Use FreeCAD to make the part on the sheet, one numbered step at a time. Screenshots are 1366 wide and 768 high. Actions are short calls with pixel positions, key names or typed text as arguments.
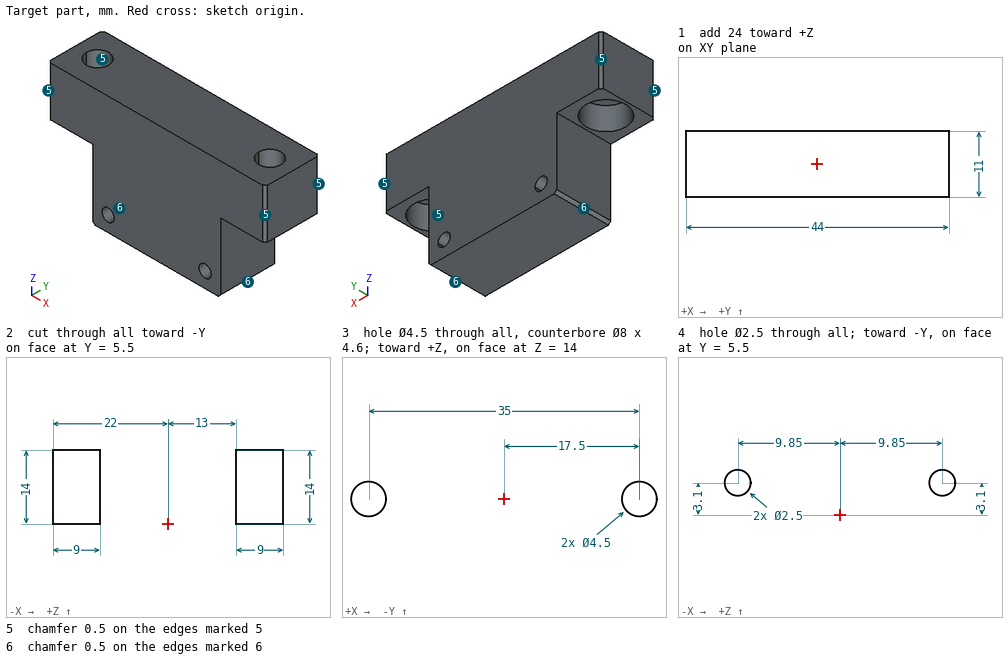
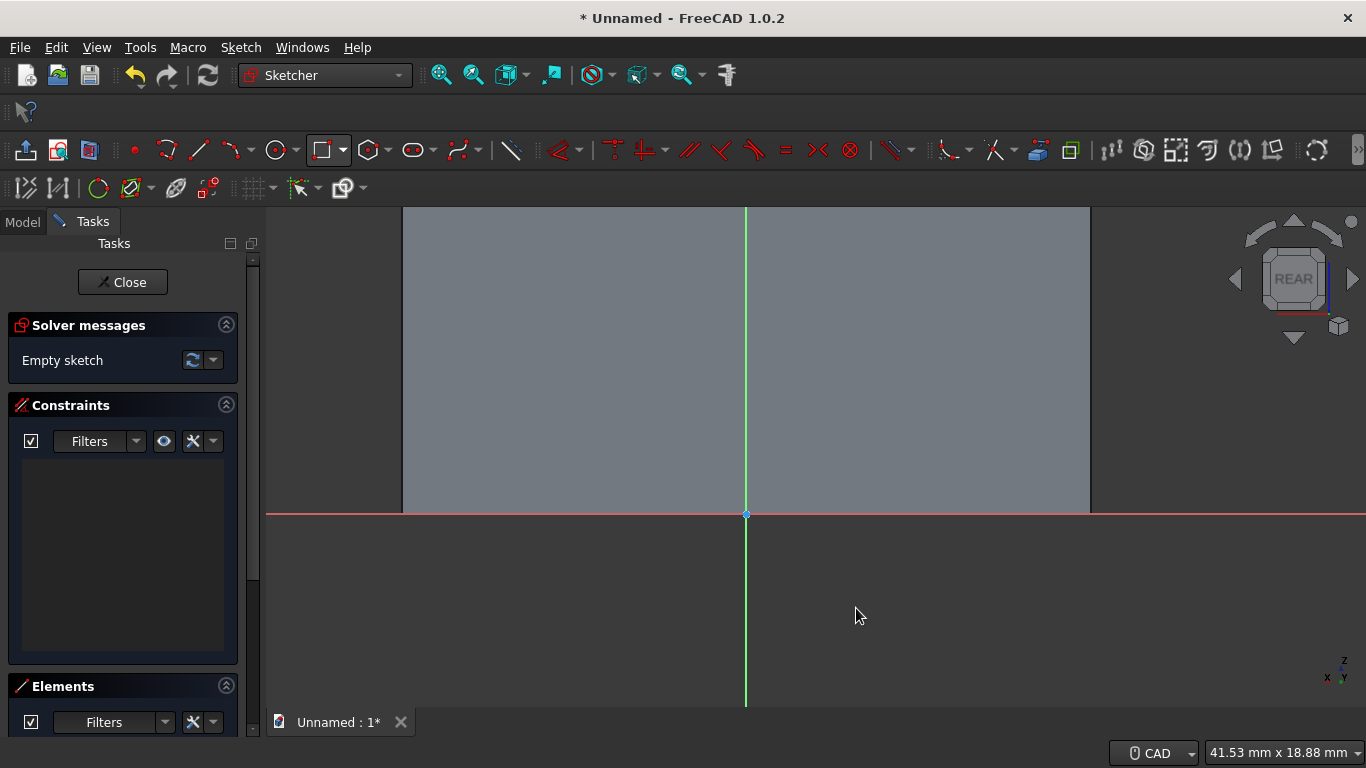
click(276, 150)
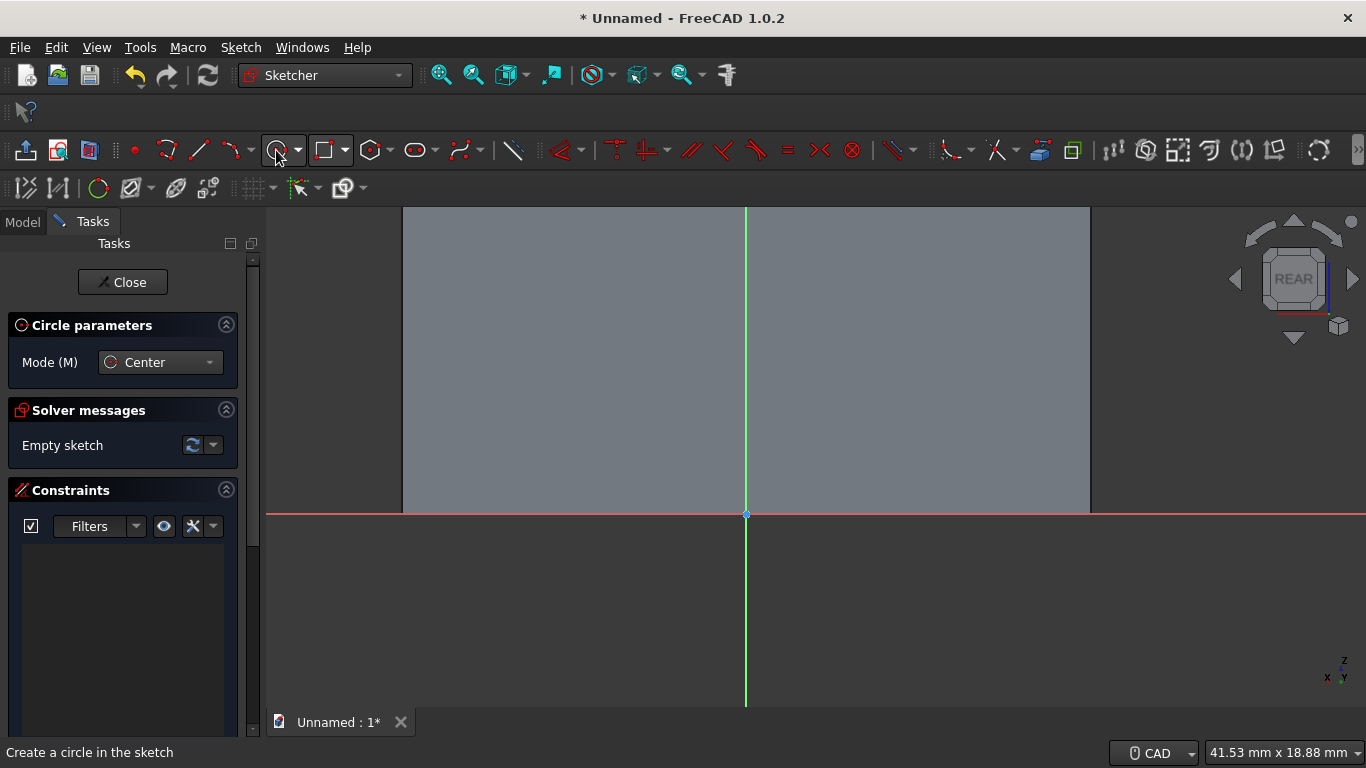
click(485, 432)
move(509, 408)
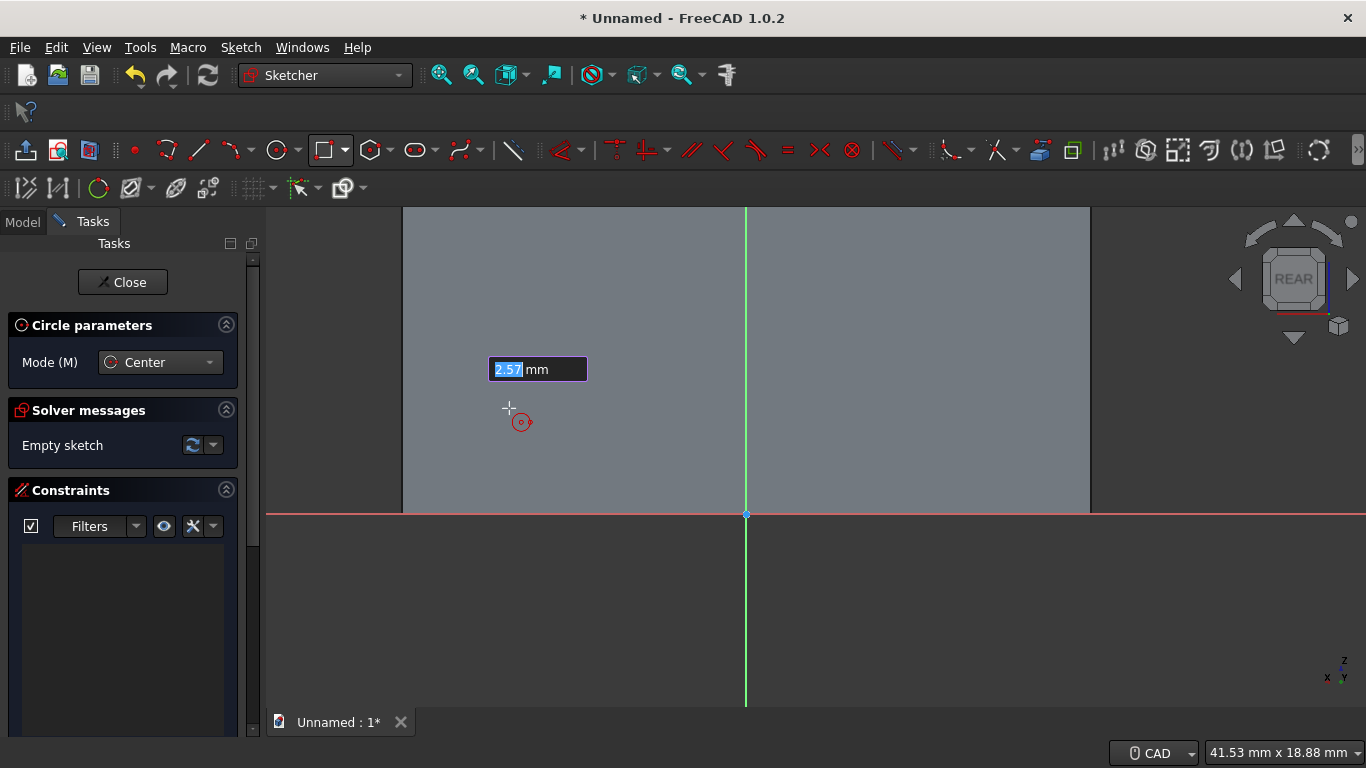
text(2.5)
key(Return)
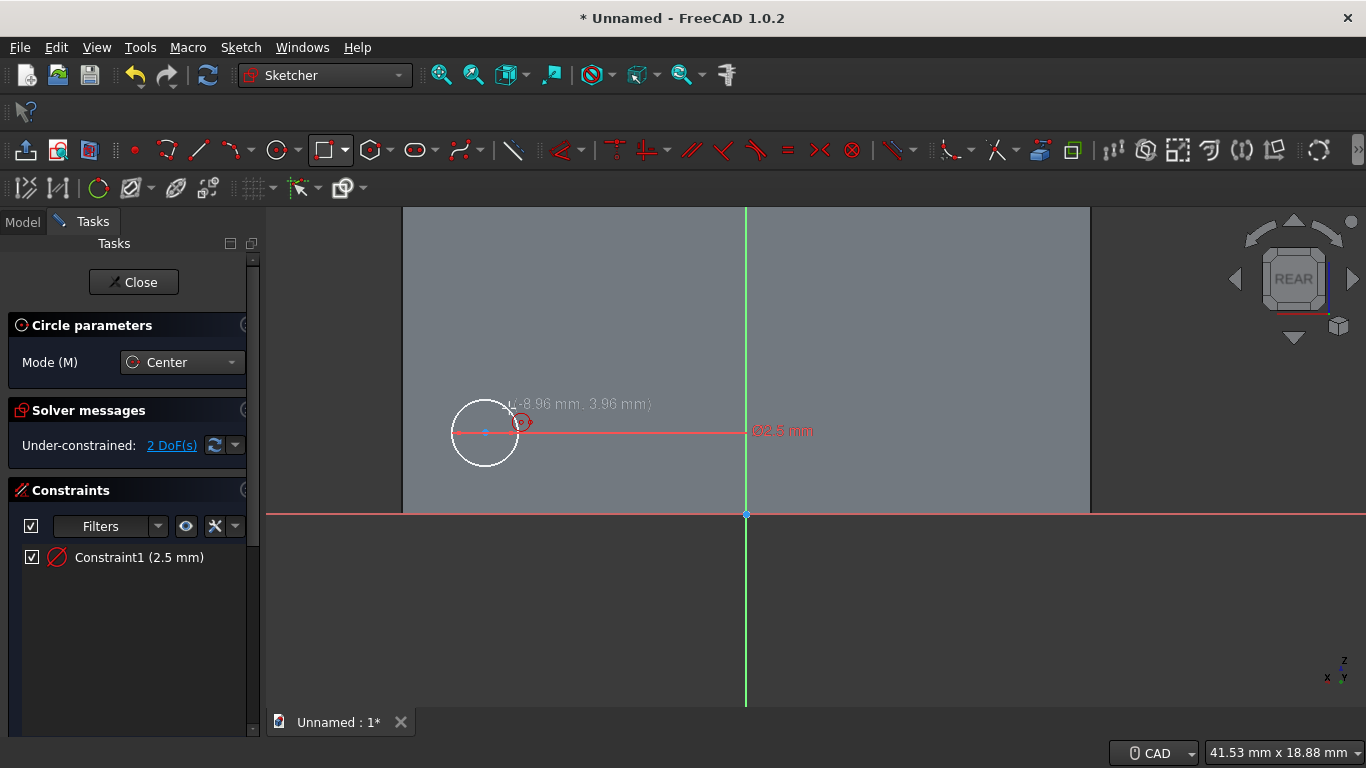
click(1007, 432)
move(1031, 408)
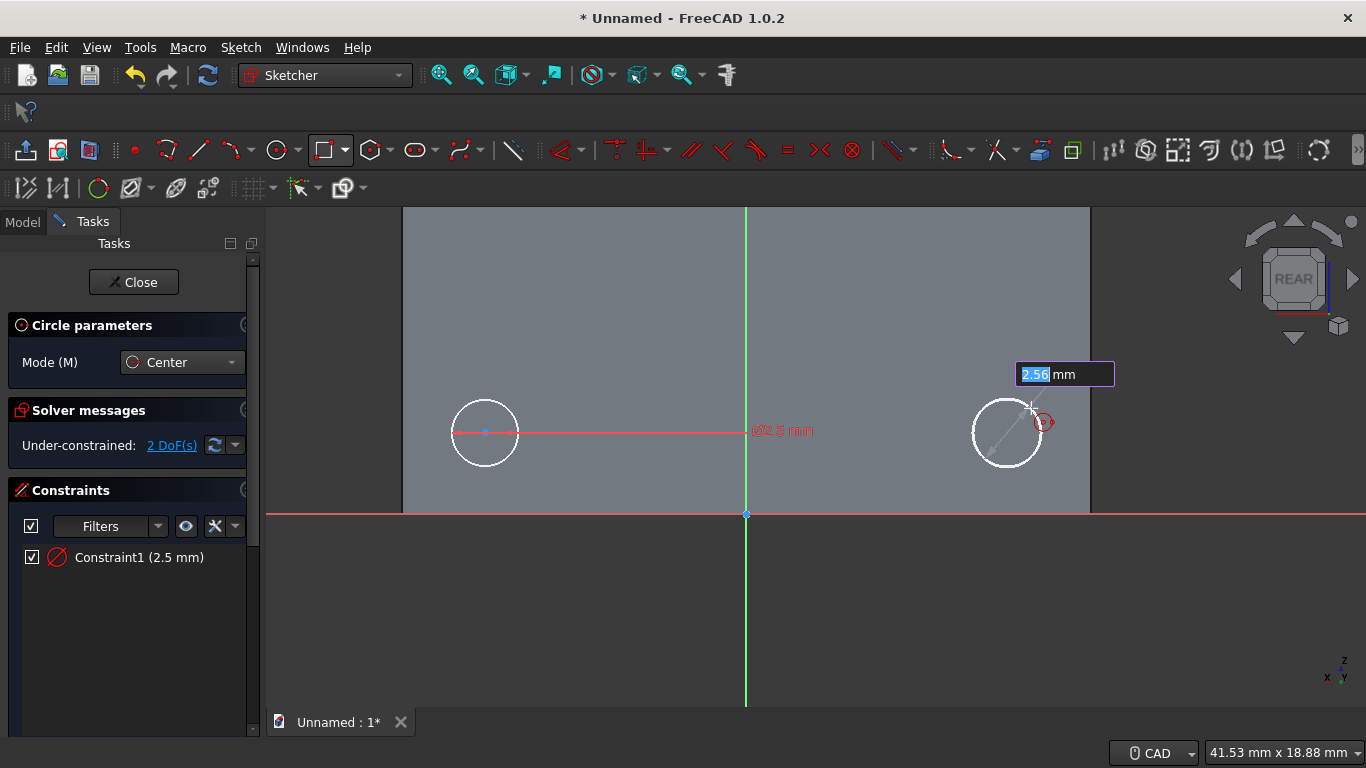
text(2.5)
key(Return)
key(Escape)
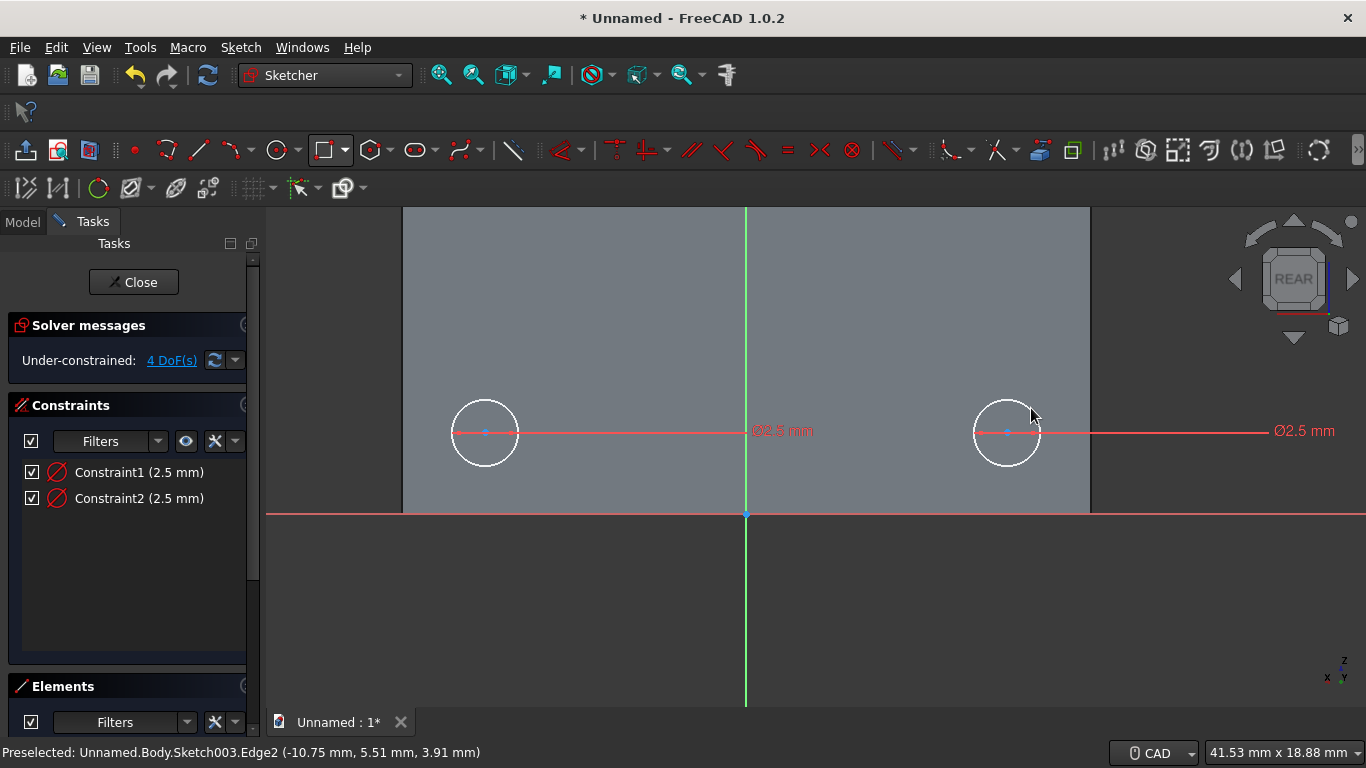
click(560, 150)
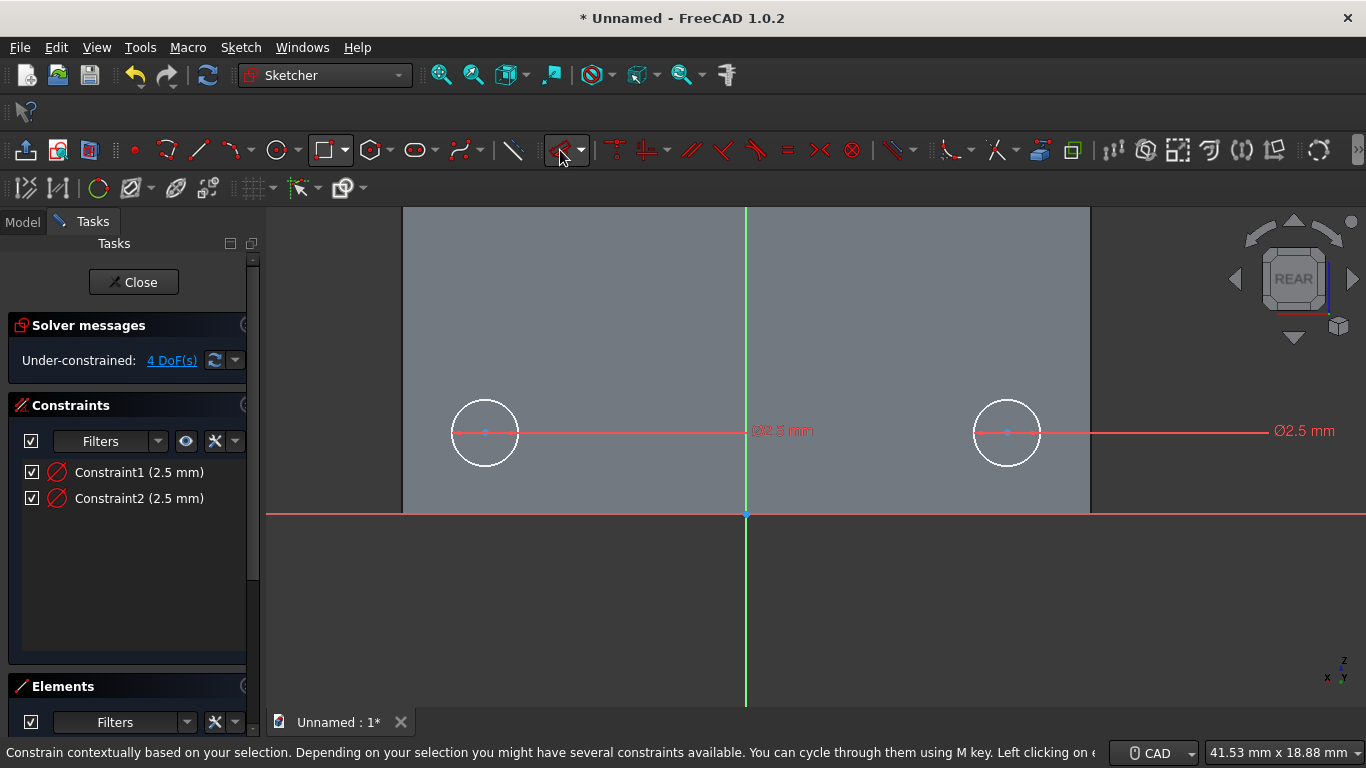
click(485, 433)
click(451, 474)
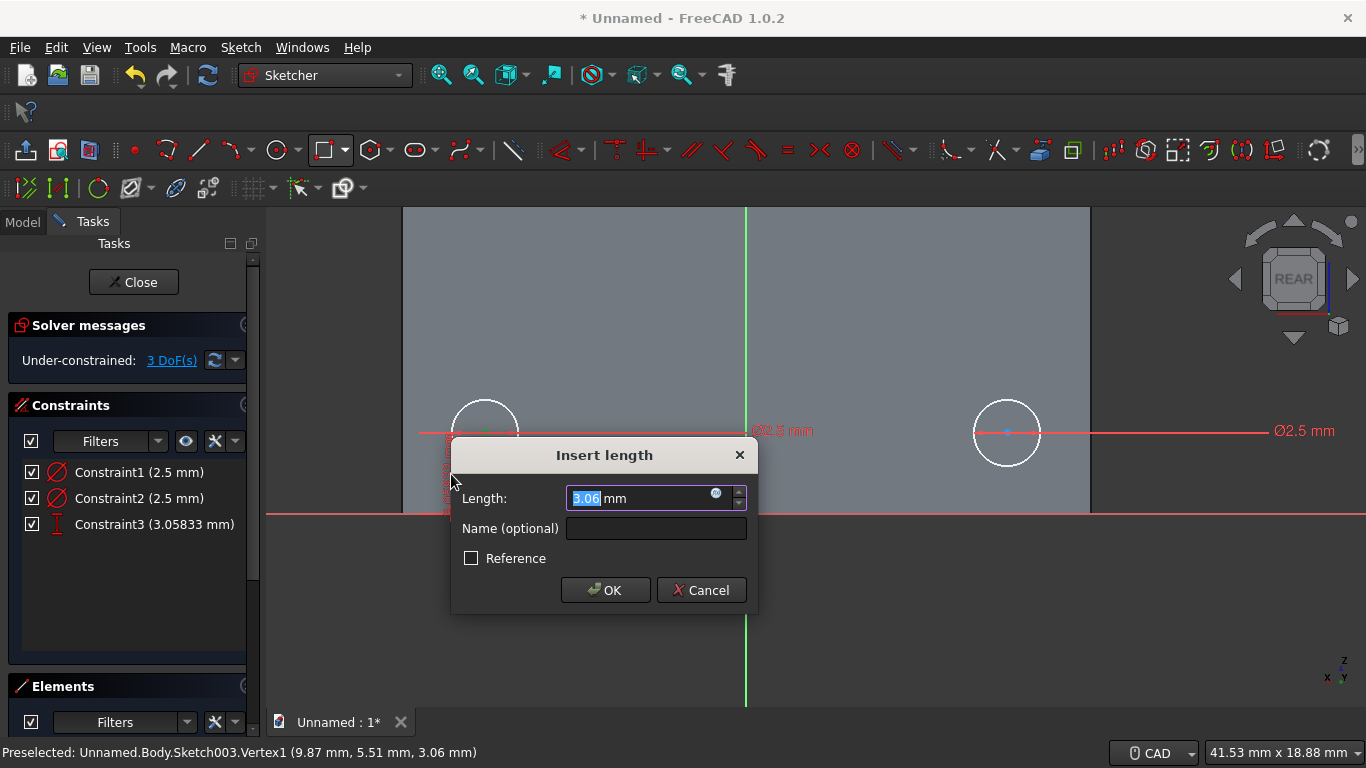
text(3.1)
key(Return)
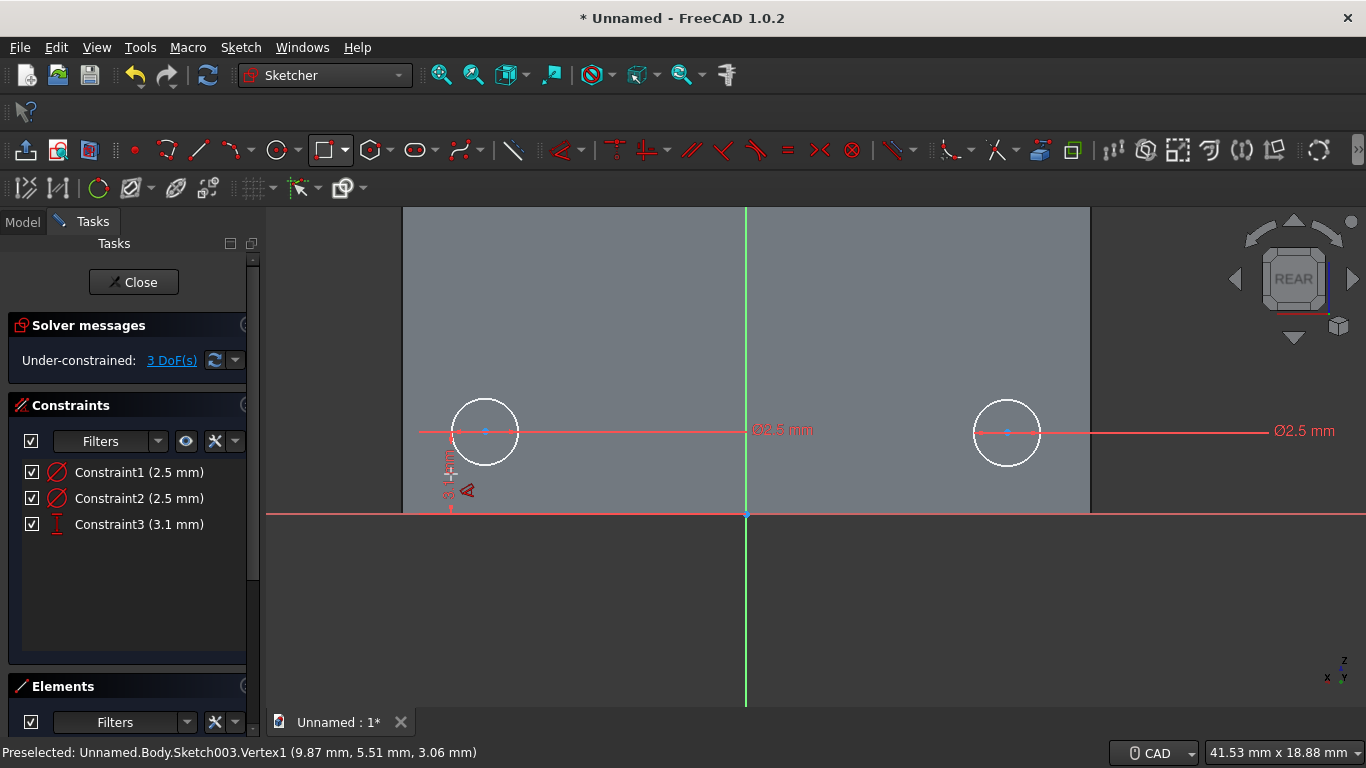
click(1007, 433)
click(1041, 474)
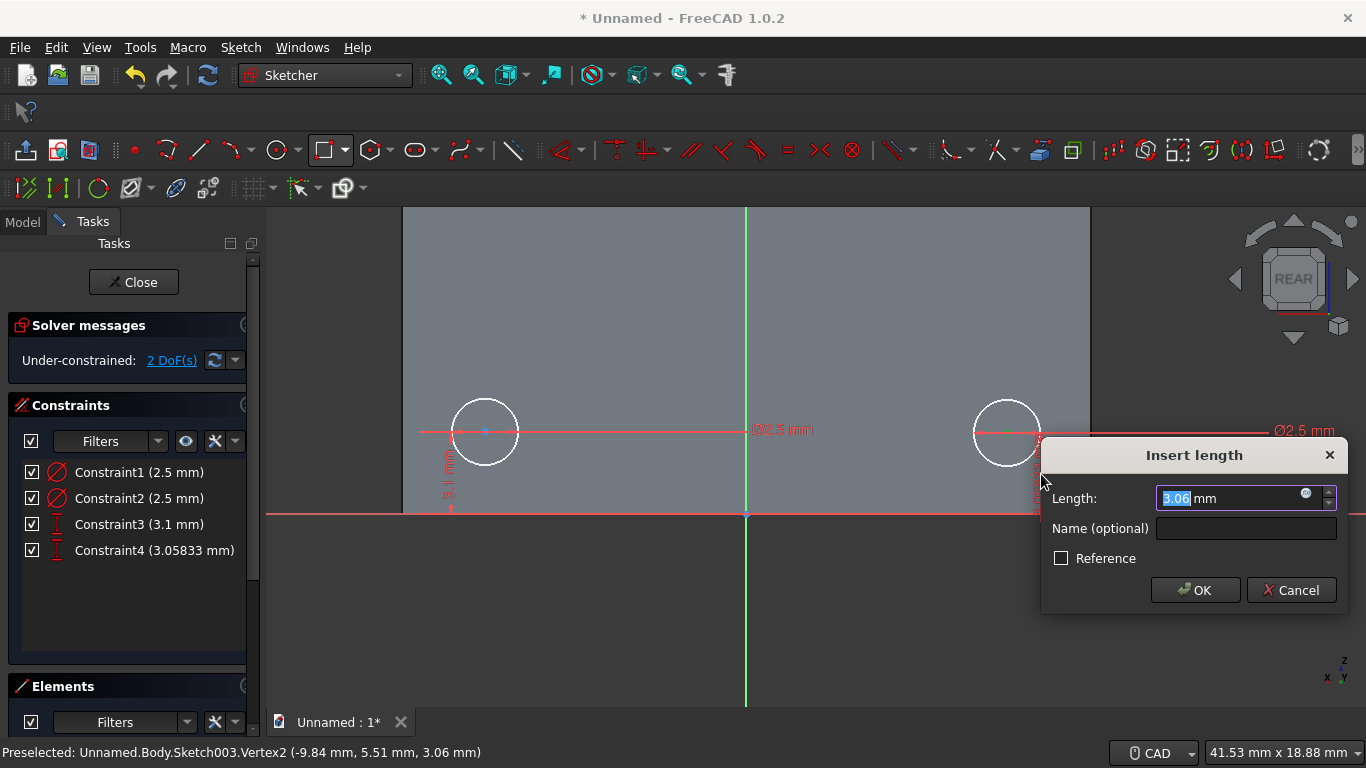
text(3.1)
key(Return)